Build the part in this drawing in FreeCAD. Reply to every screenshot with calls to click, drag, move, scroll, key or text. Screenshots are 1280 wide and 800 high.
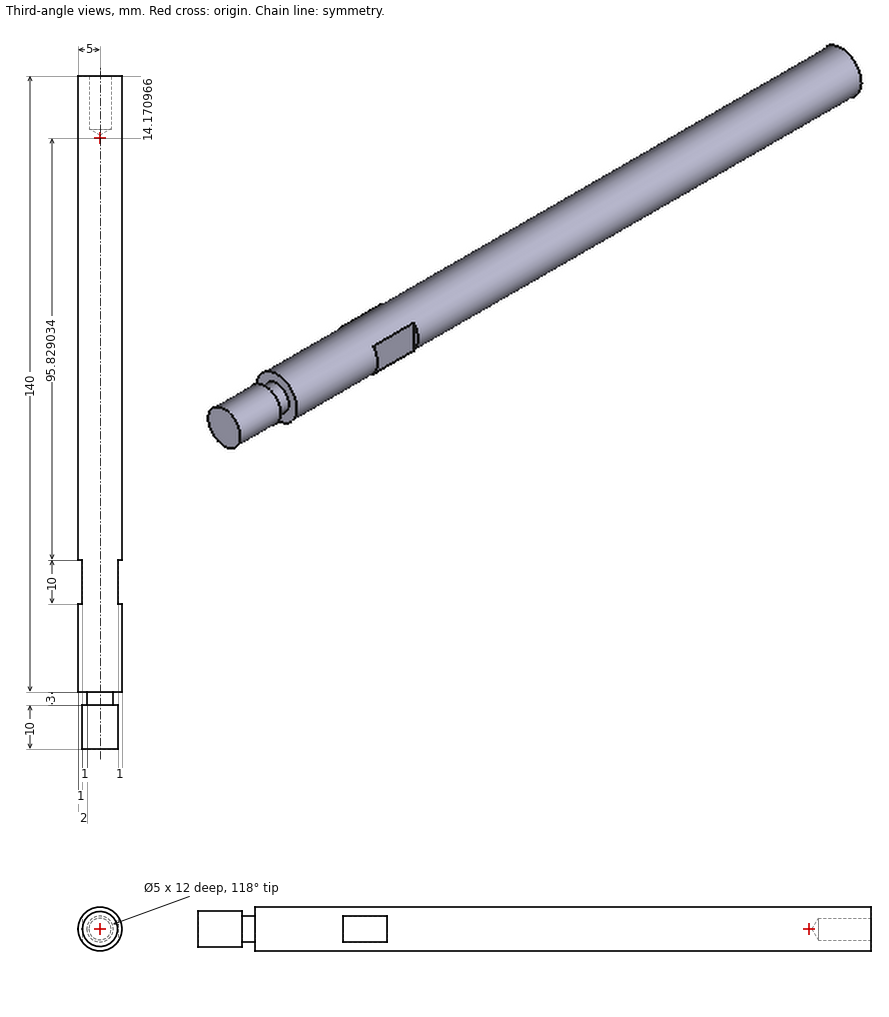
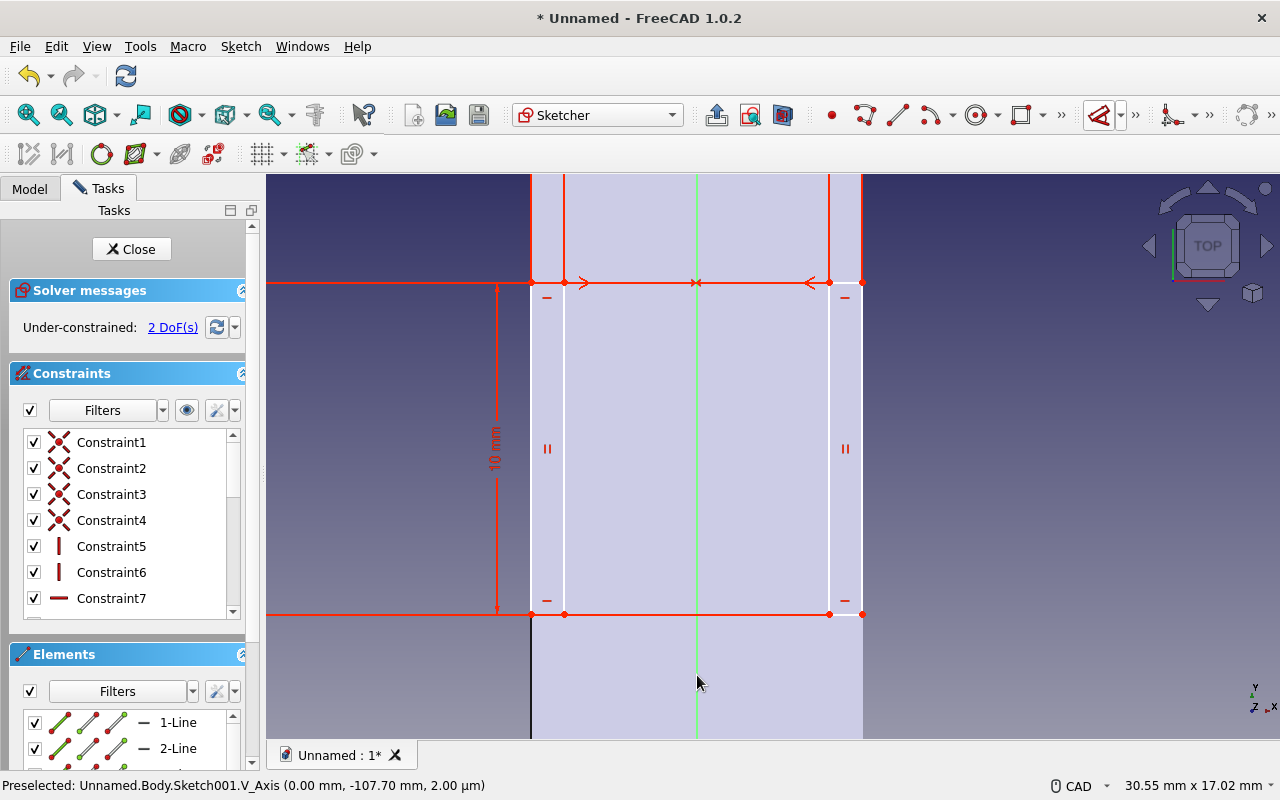
click(531, 283)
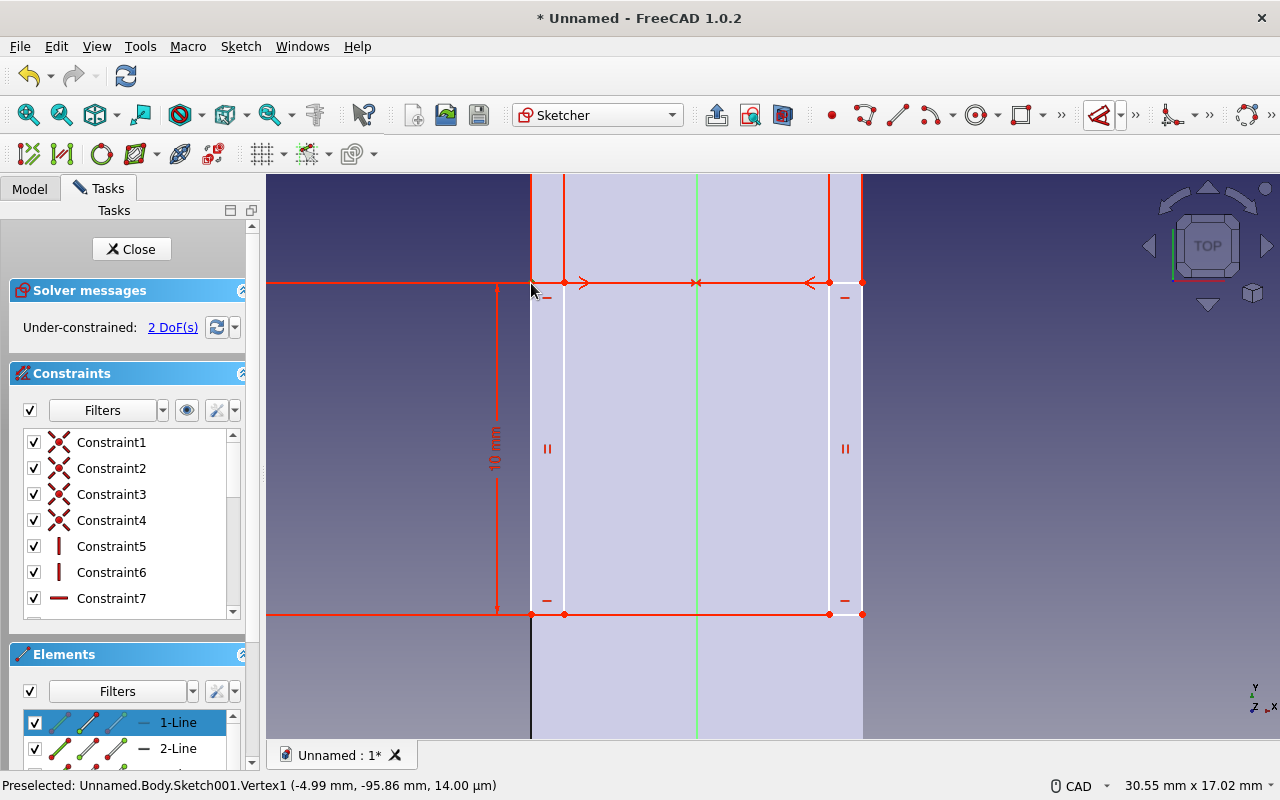
key(l)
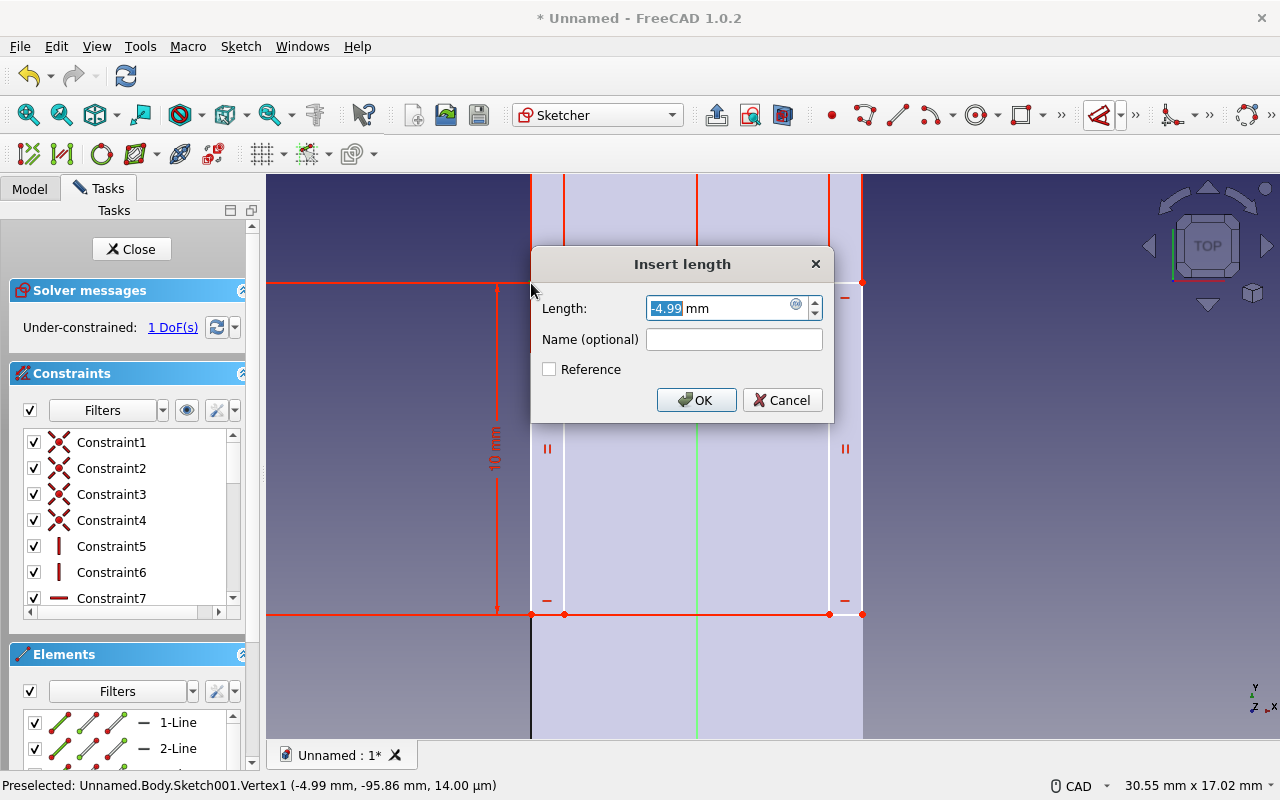
text(-5)
key(Return)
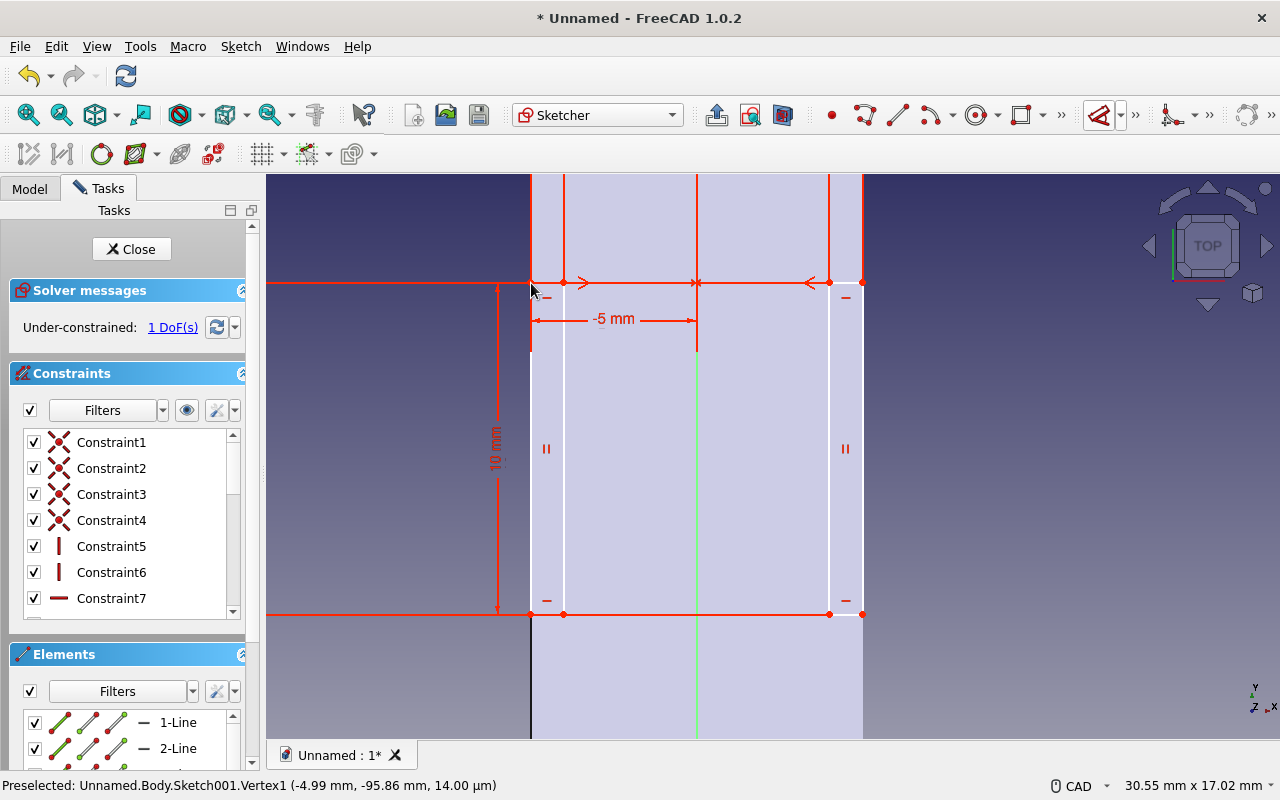
click(531, 283)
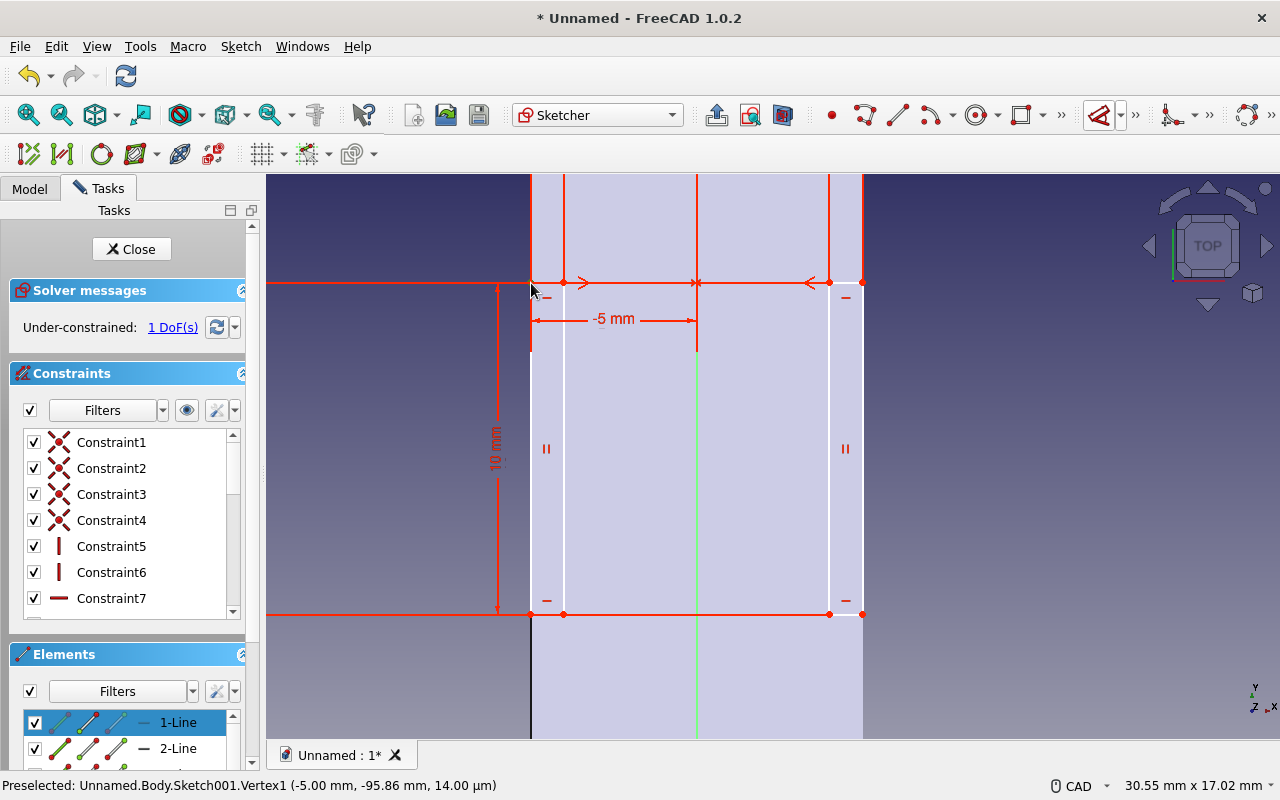
key(i)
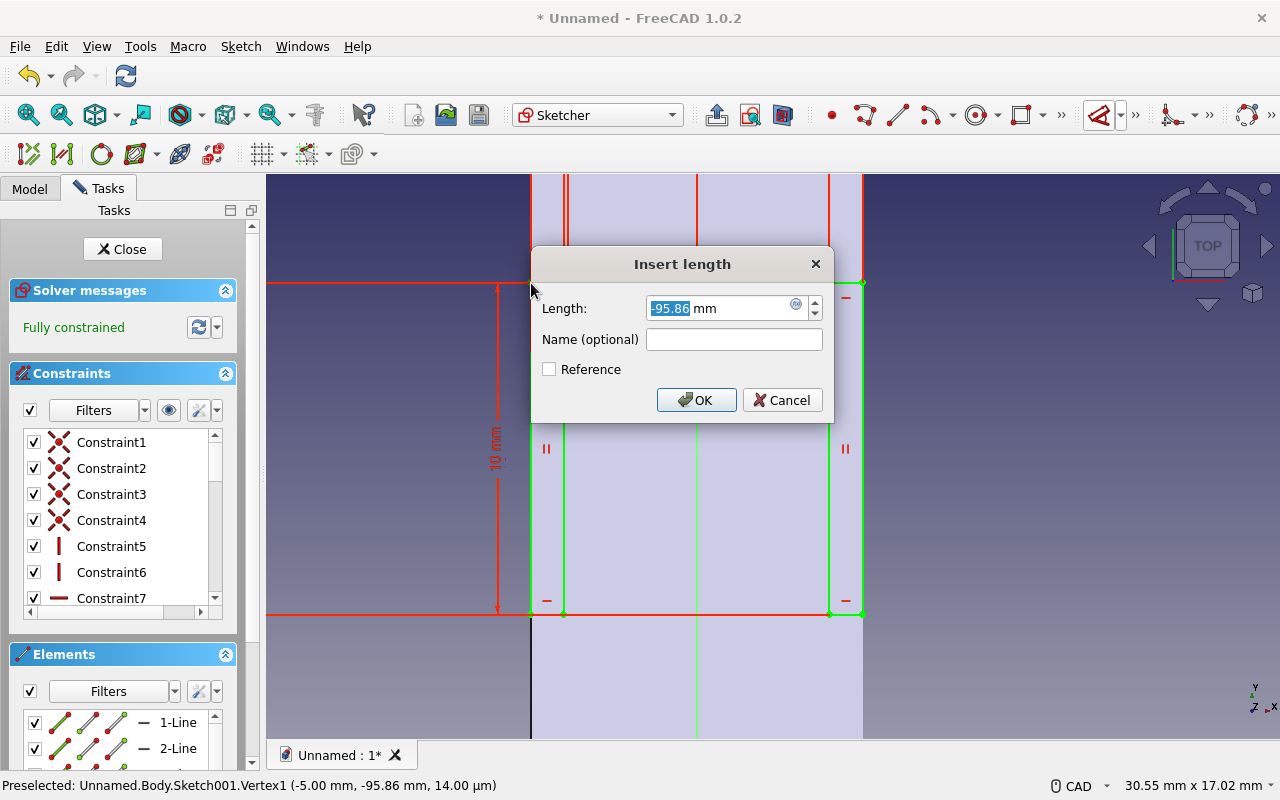
text(-95.829034)
key(Return)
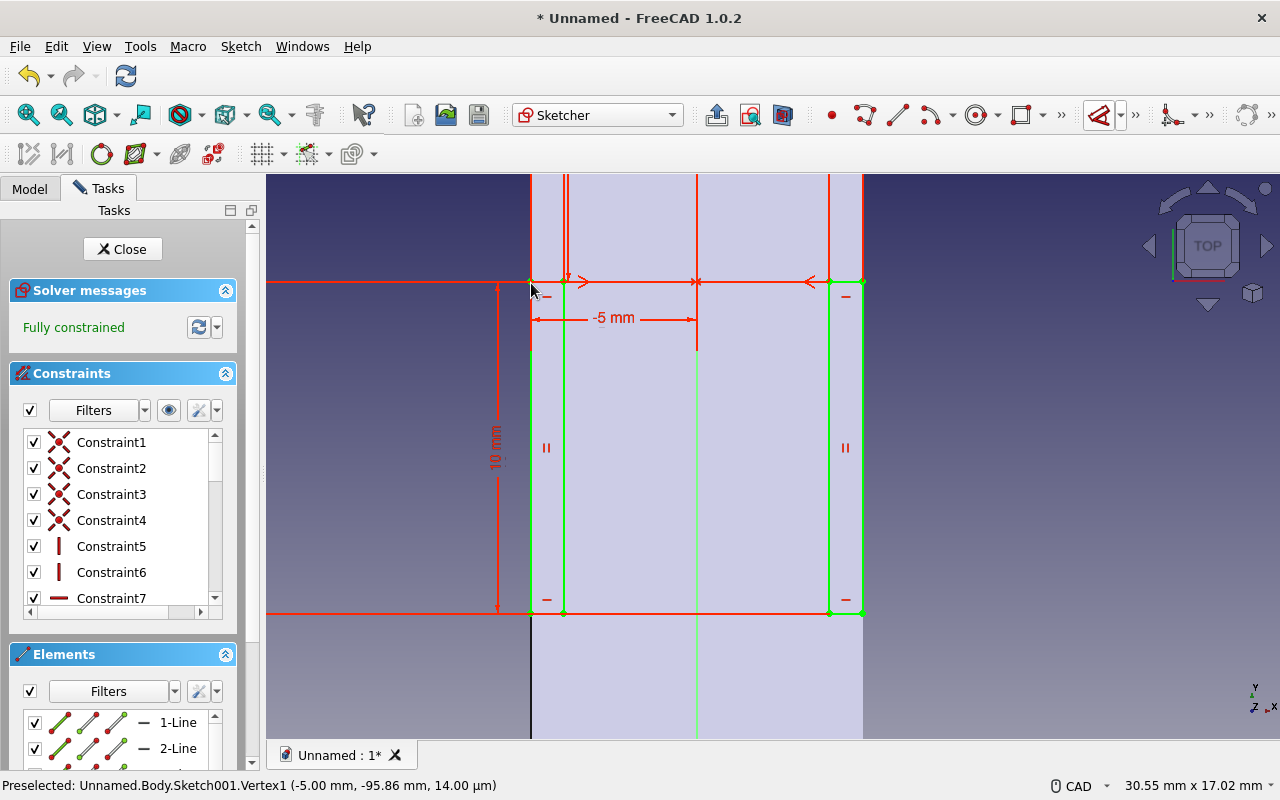
click(123, 249)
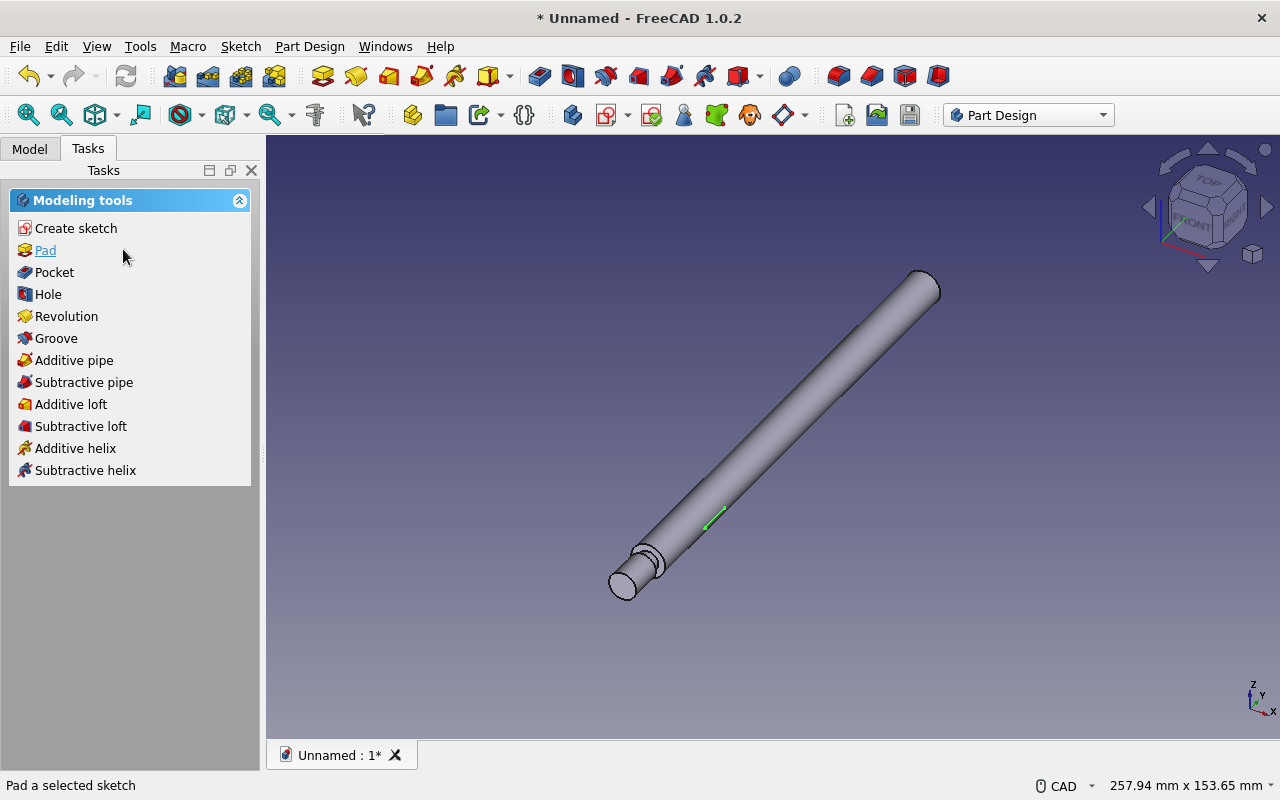
click(540, 76)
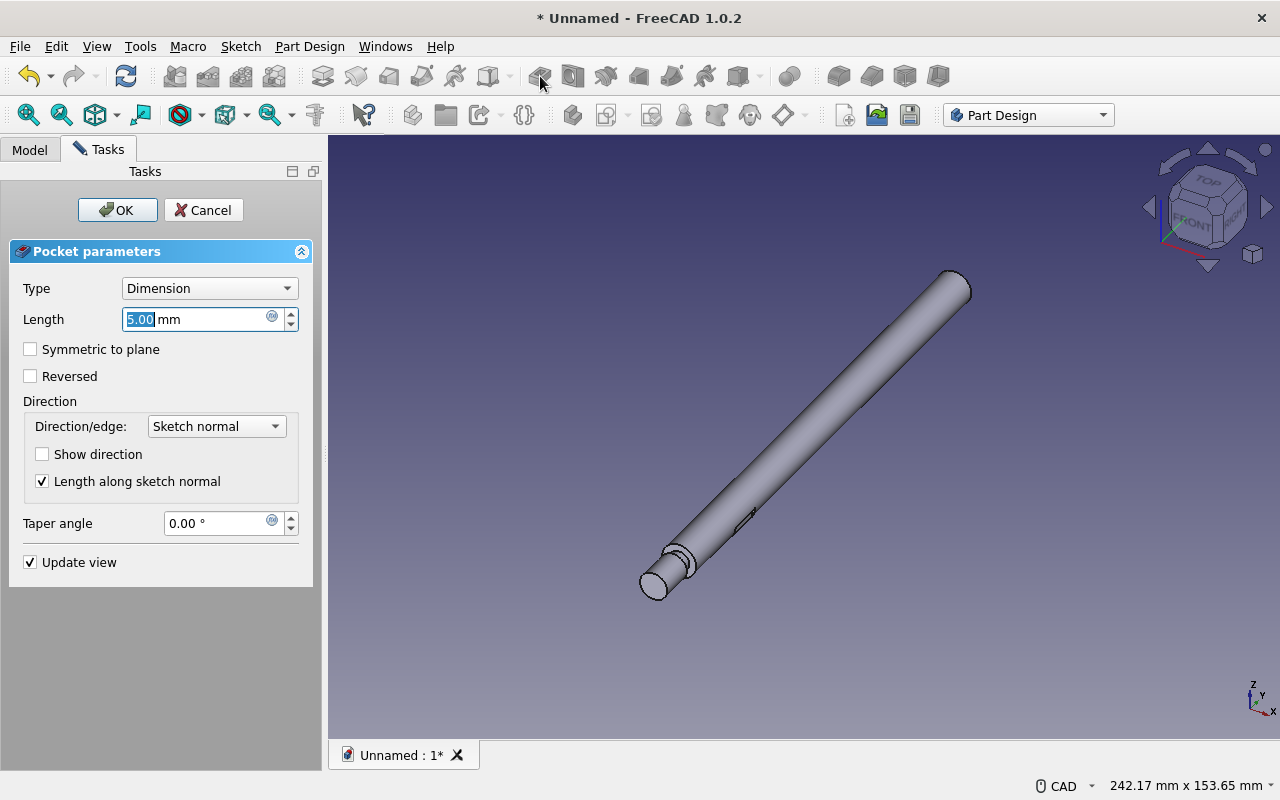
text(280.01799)
key(Tab)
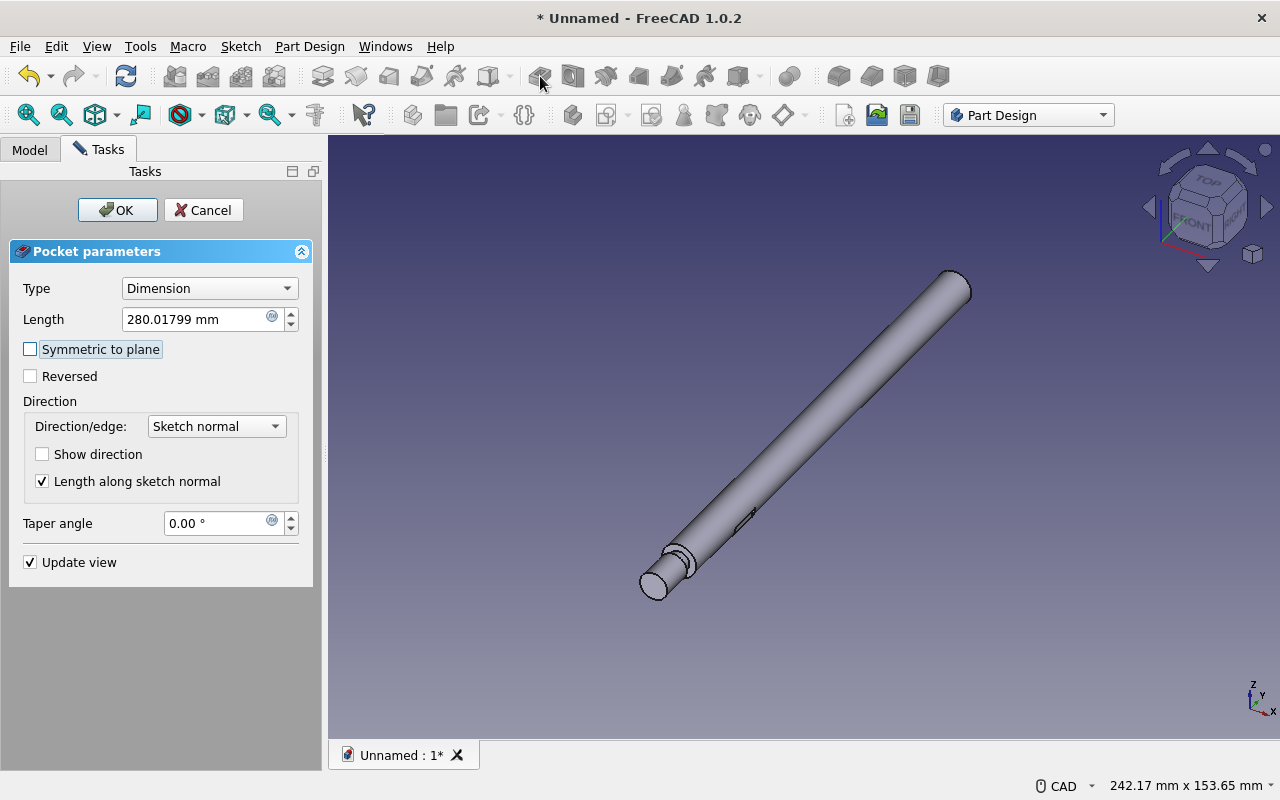
click(31, 349)